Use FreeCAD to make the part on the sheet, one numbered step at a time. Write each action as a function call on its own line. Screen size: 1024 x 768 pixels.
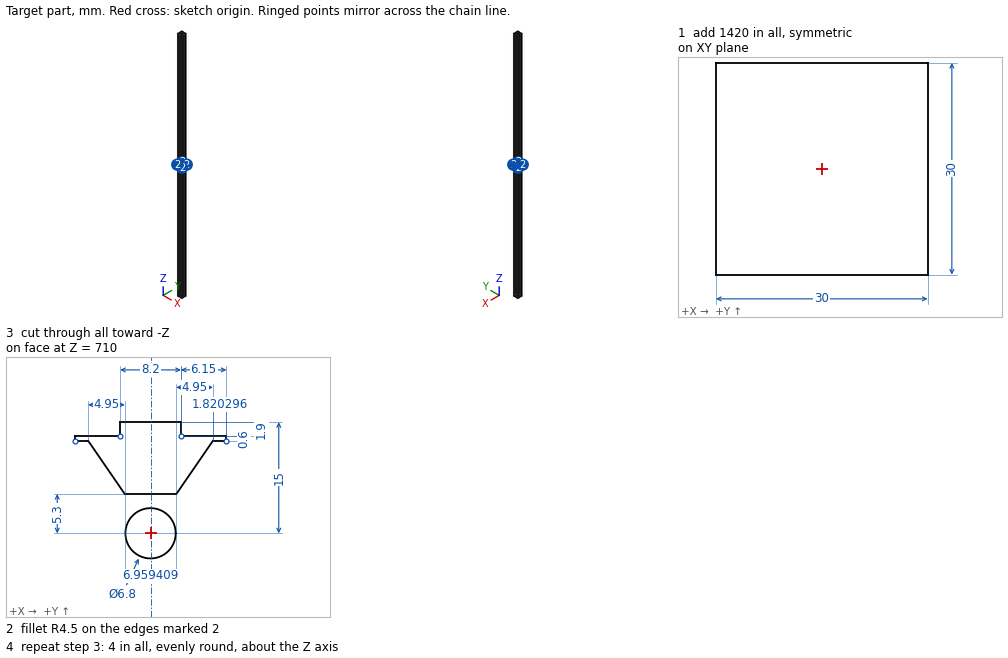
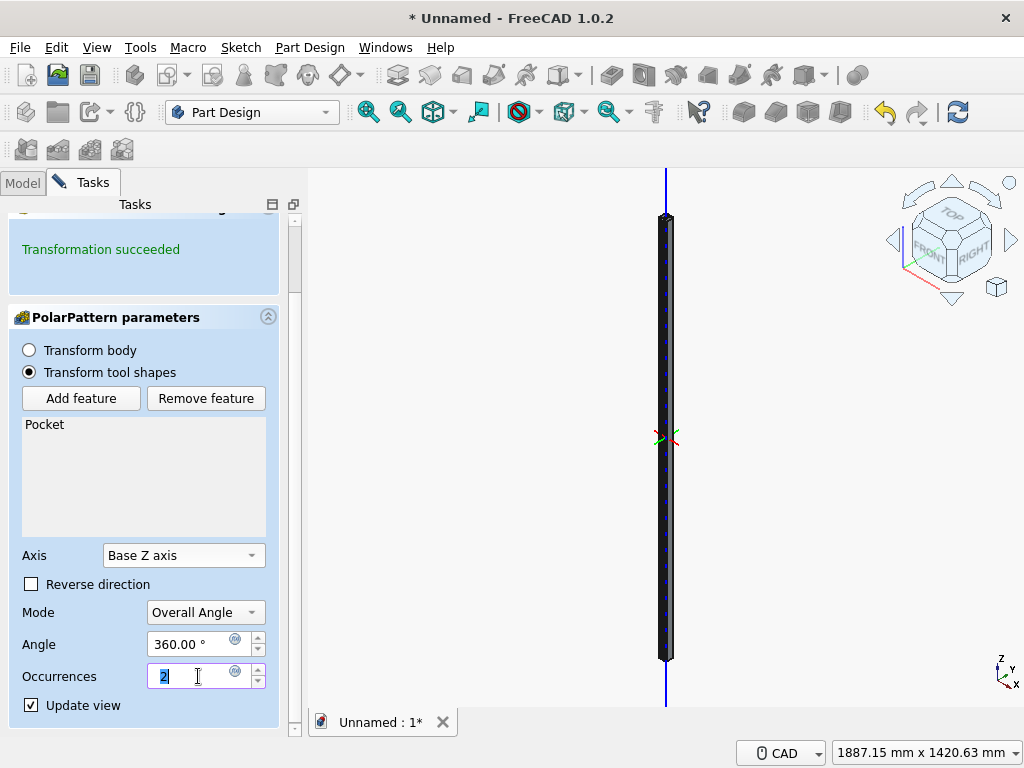
text(4)
key(Tab)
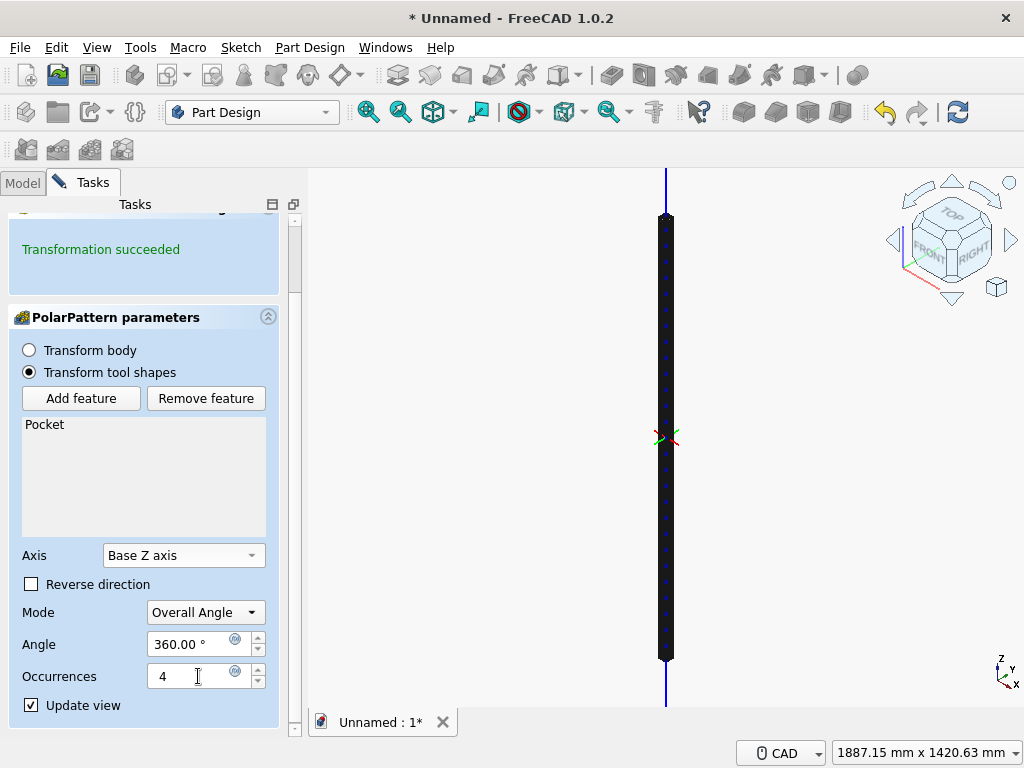
scroll(295, 475, up, 3)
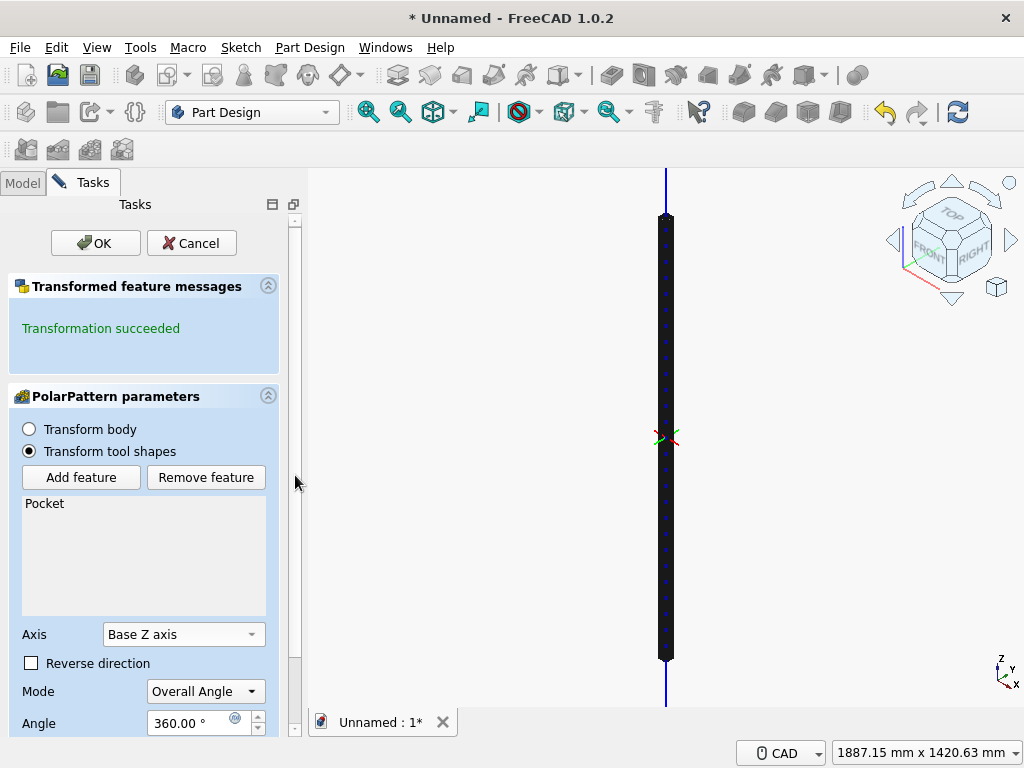
click(96, 243)